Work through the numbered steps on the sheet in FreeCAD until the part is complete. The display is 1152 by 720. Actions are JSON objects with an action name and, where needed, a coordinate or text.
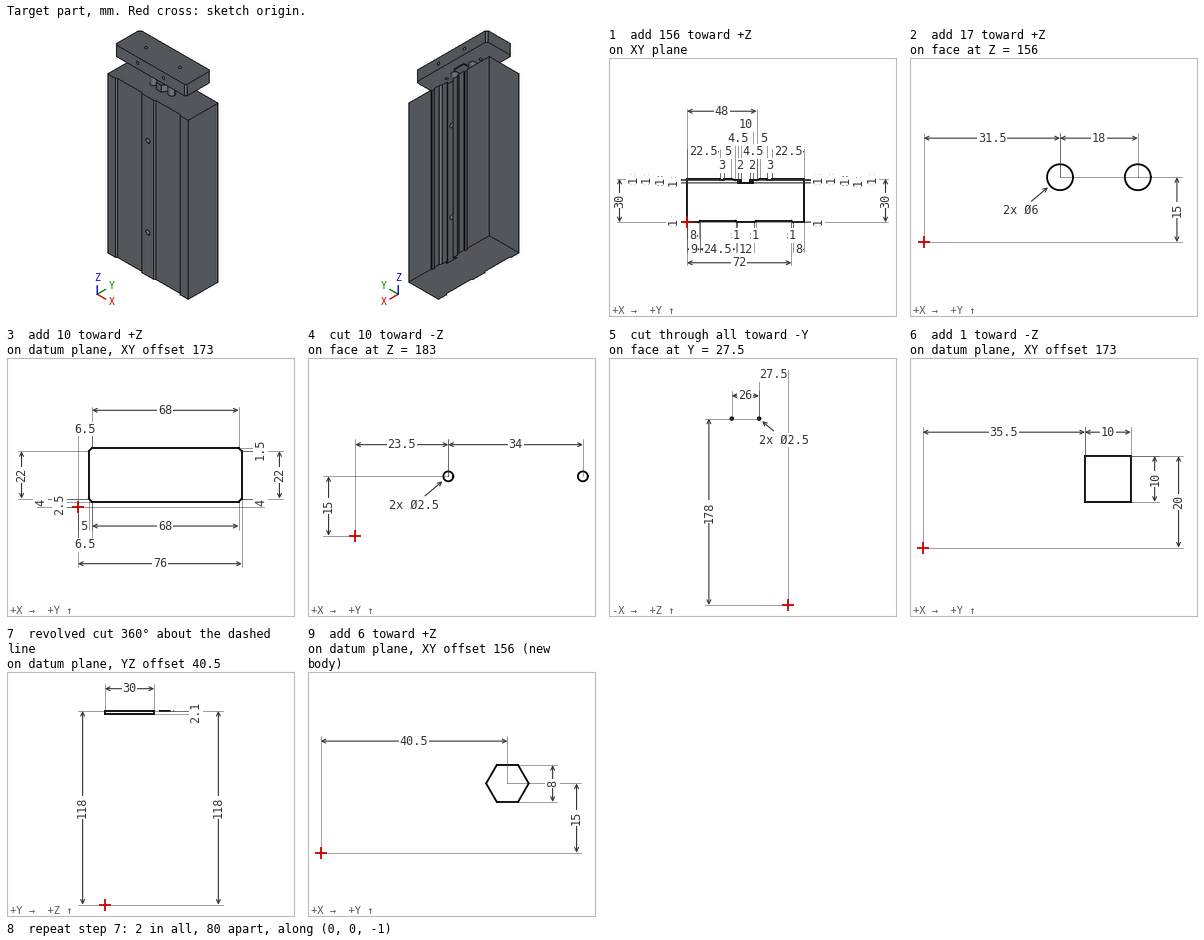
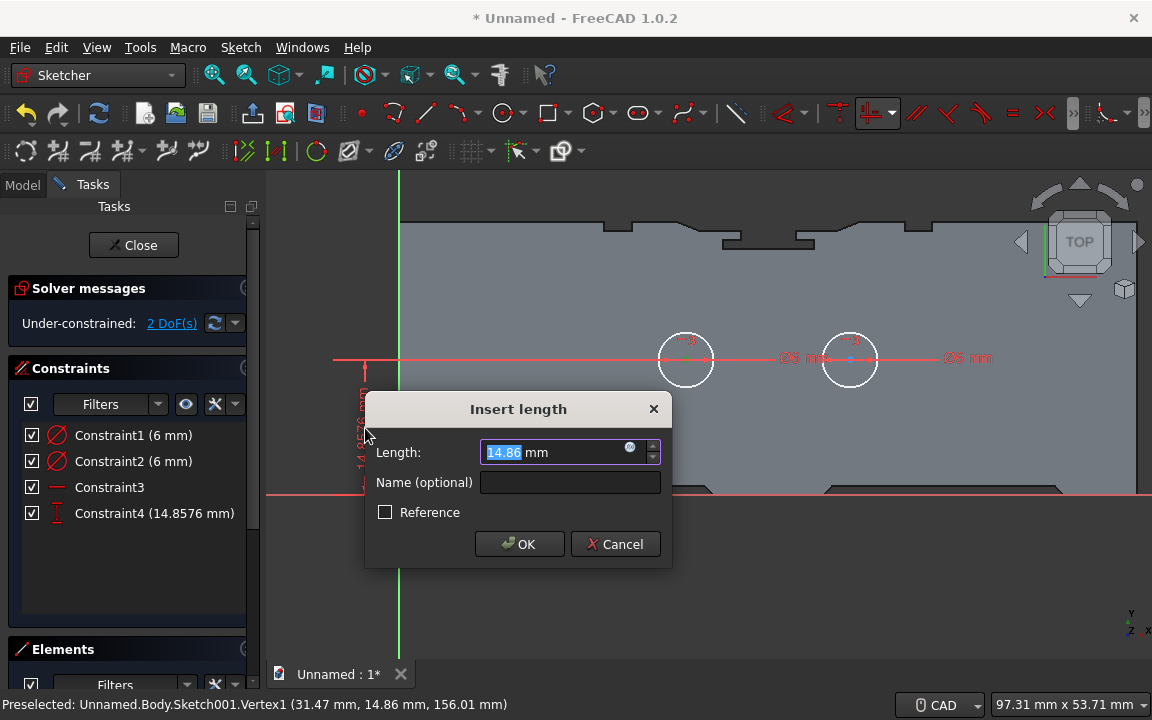
{"action": "type", "text": "15"}
{"action": "key", "text": "Return"}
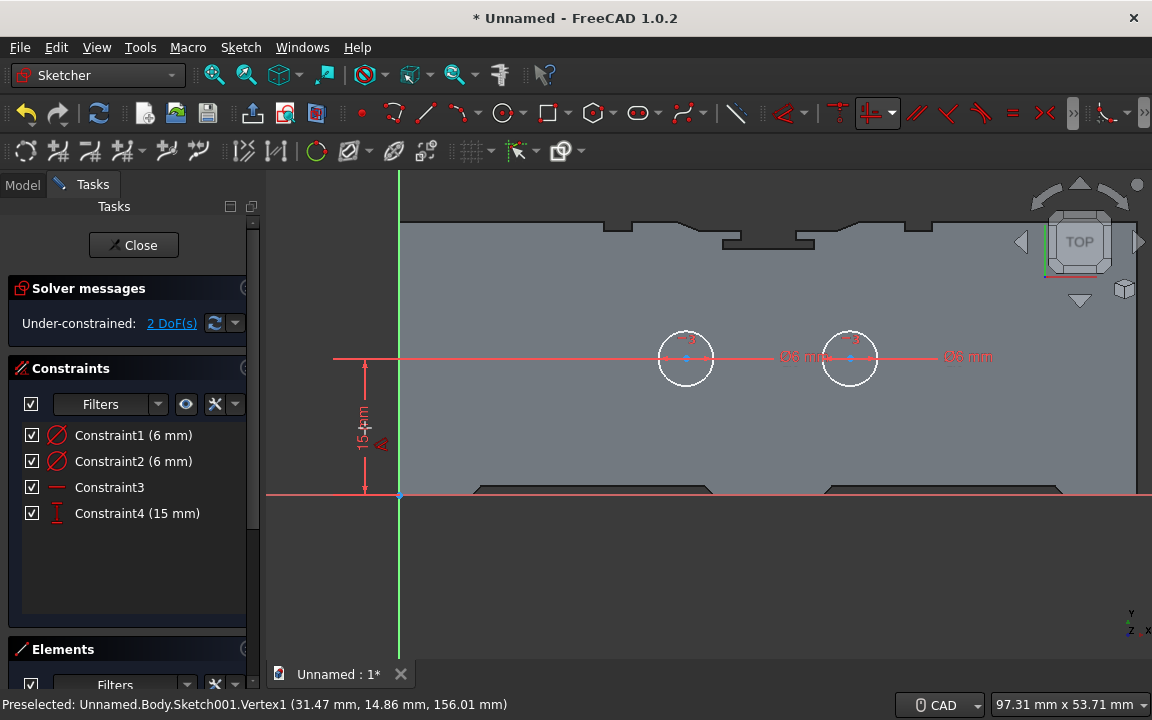
{"action": "left_click", "coordinate": [686, 359]}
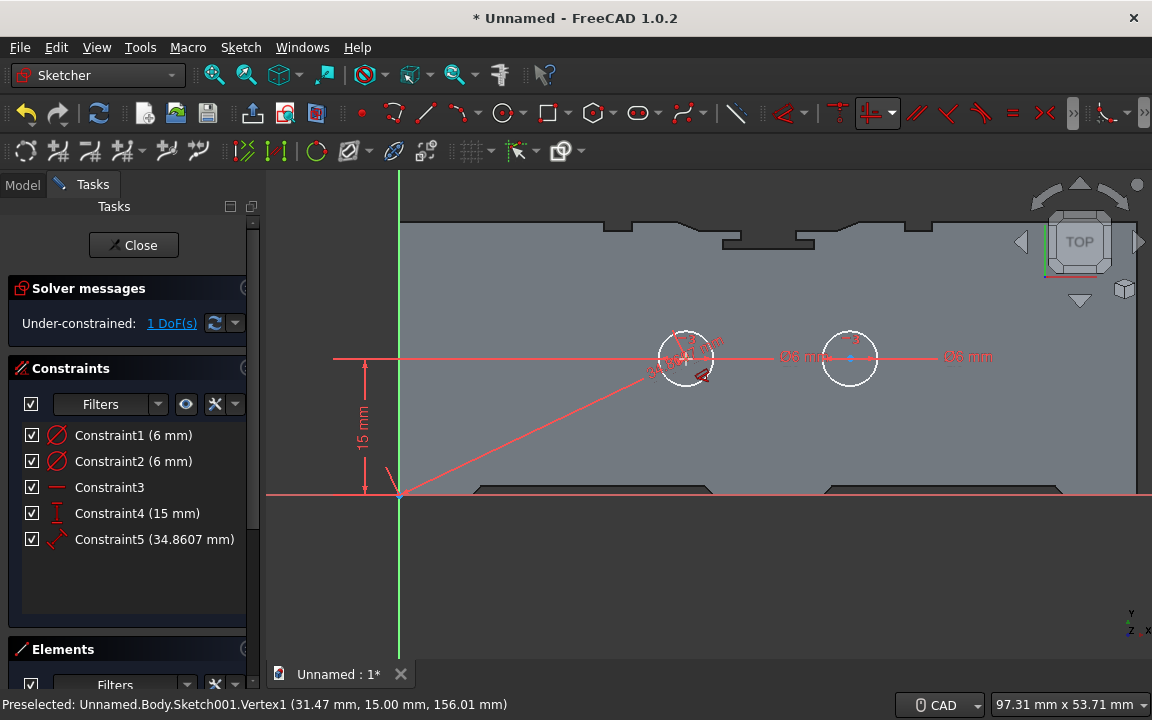
{"action": "left_click", "coordinate": [850, 359]}
{"action": "left_click", "coordinate": [768, 325]}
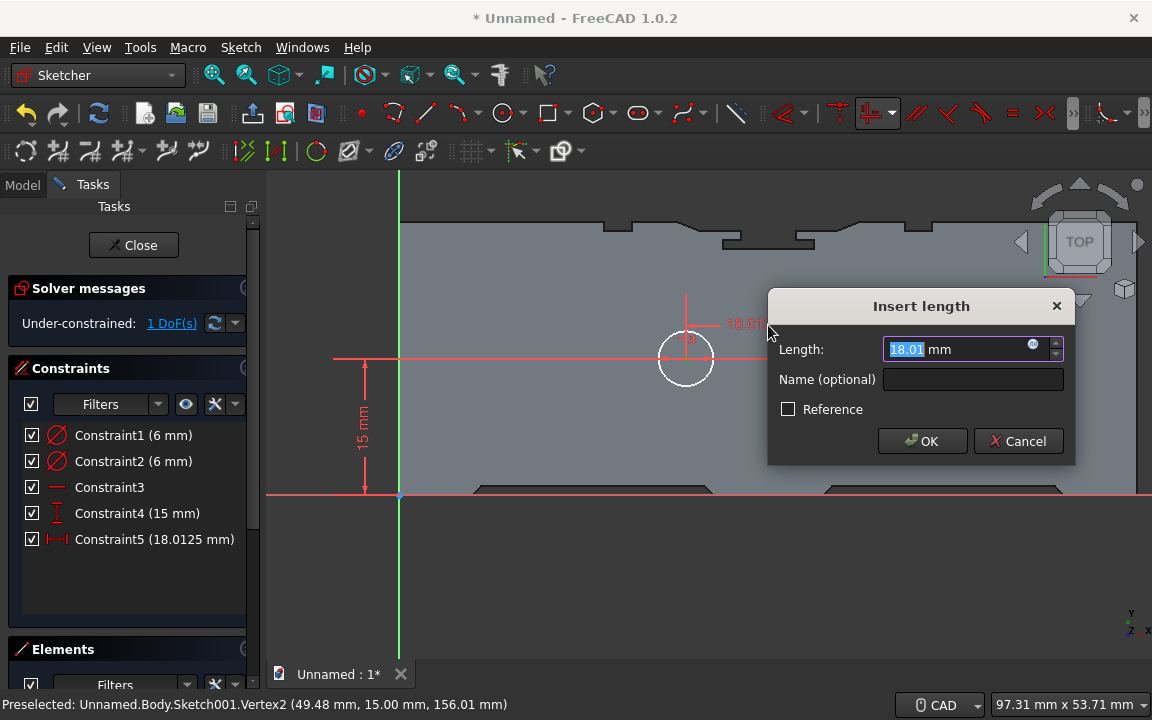
{"action": "type", "text": "18"}
{"action": "key", "text": "Return"}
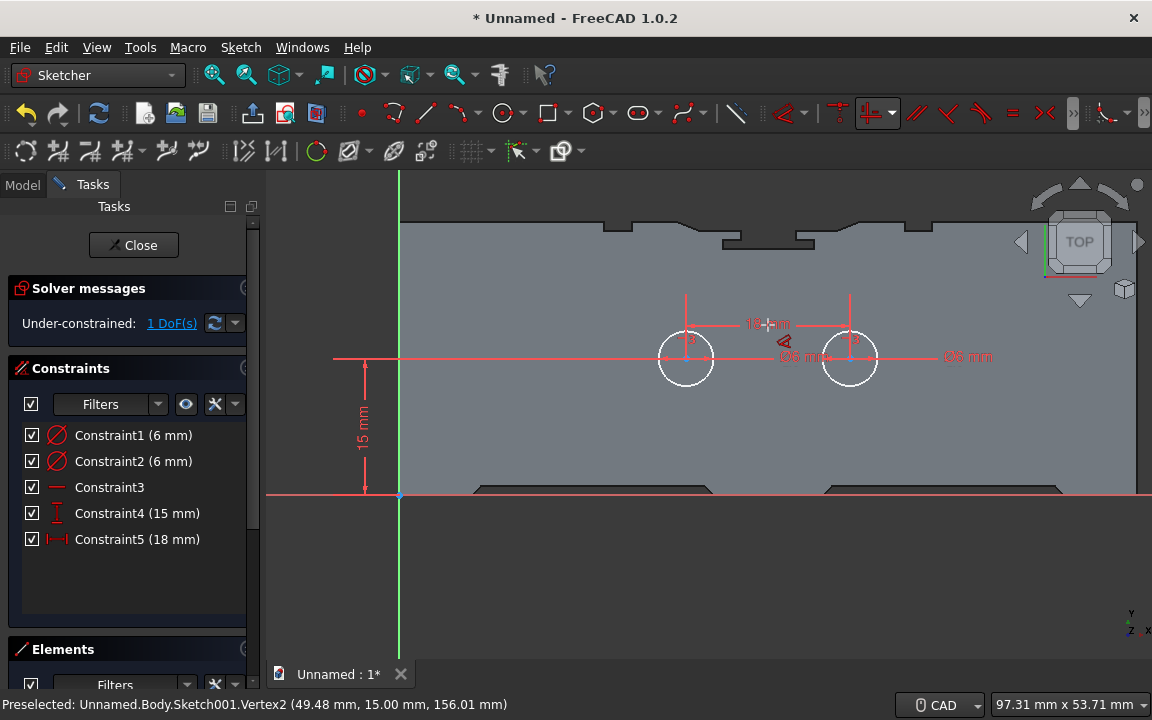
{"action": "left_click", "coordinate": [686, 359]}
{"action": "left_click", "coordinate": [543, 529]}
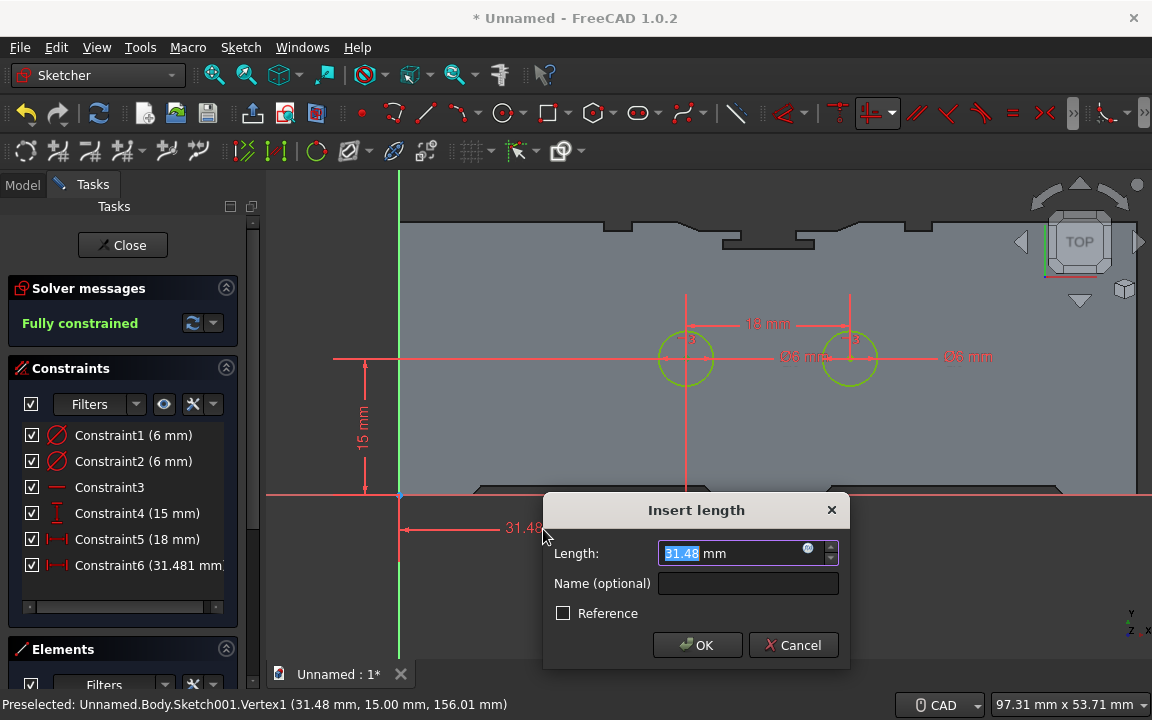
{"action": "type", "text": "31.5"}
{"action": "key", "text": "Return"}
{"action": "key", "text": "Escape"}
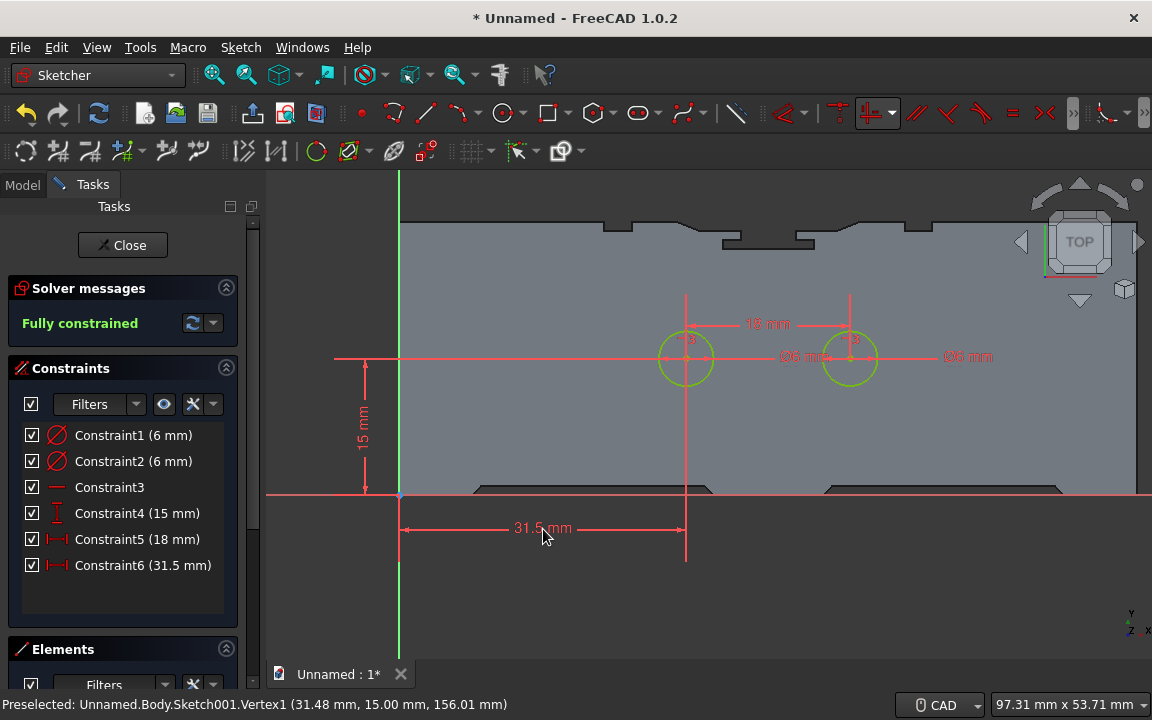
{"action": "left_click", "coordinate": [123, 245]}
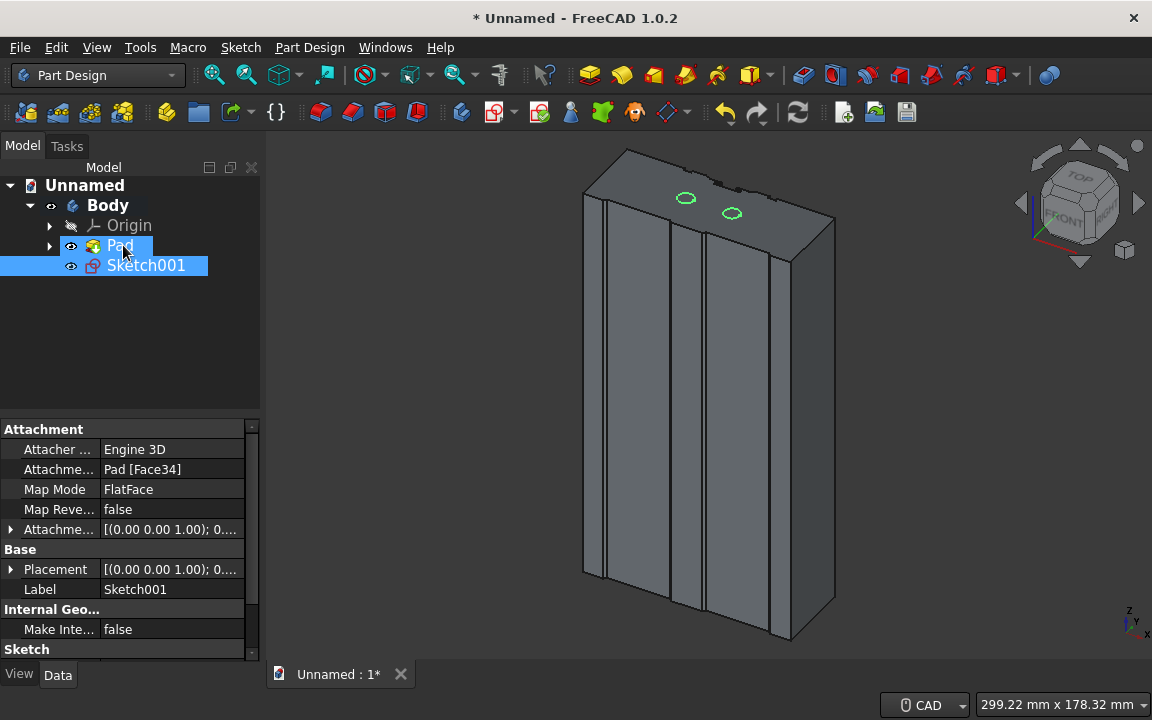
{"action": "left_click", "coordinate": [590, 76]}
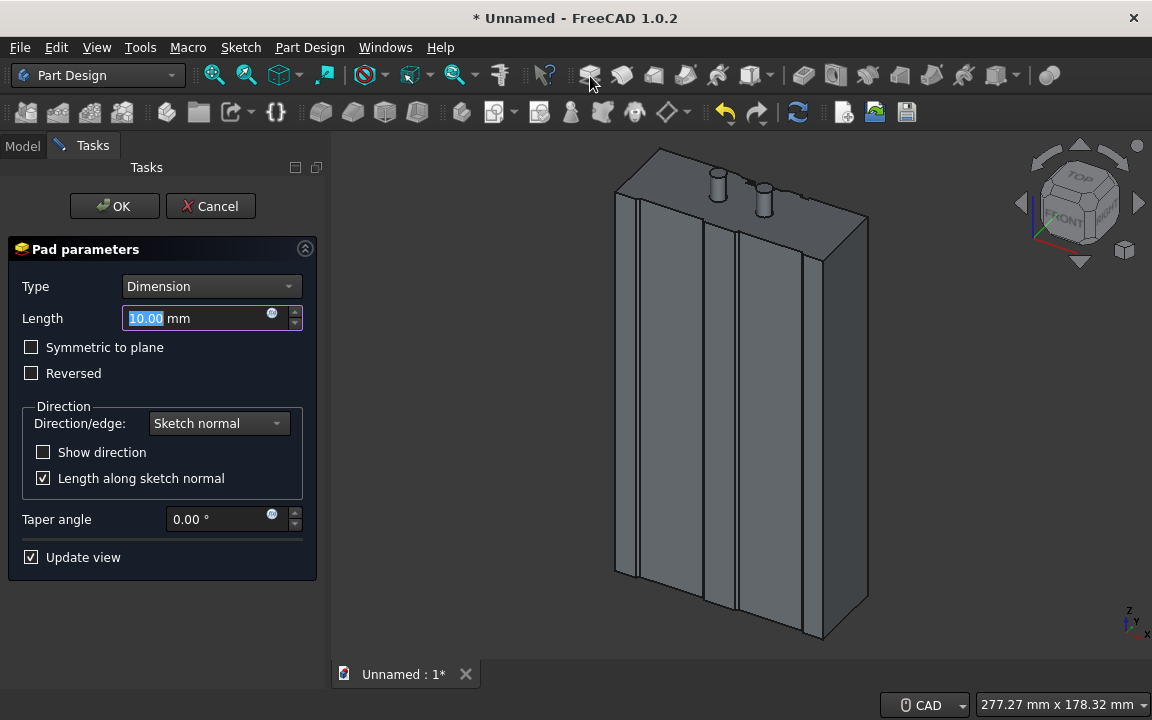
{"action": "type", "text": "17"}
{"action": "key", "text": "Tab"}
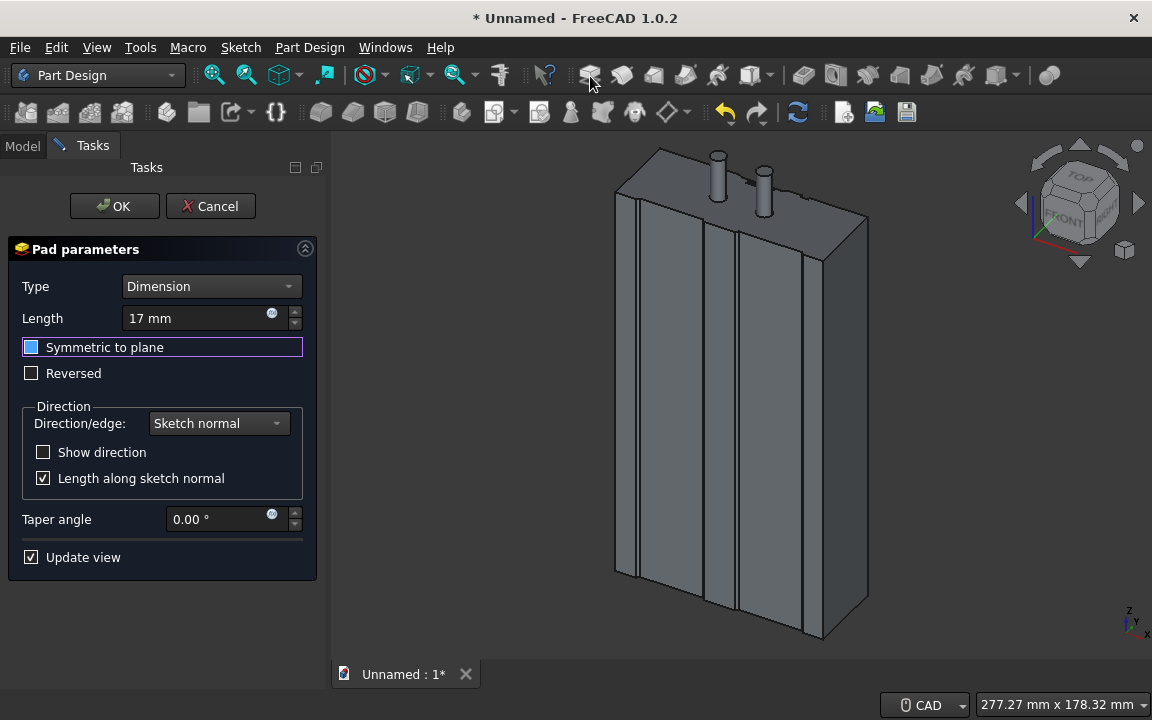
{"action": "left_click", "coordinate": [115, 206]}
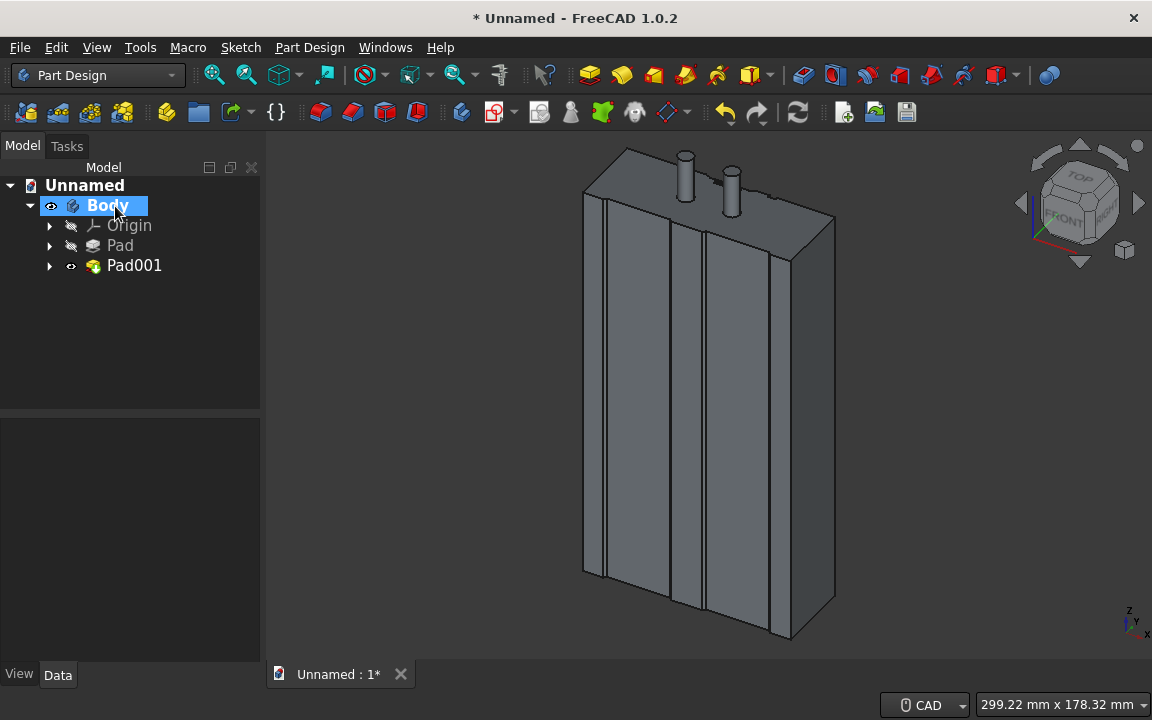
{"action": "key", "text": "v f"}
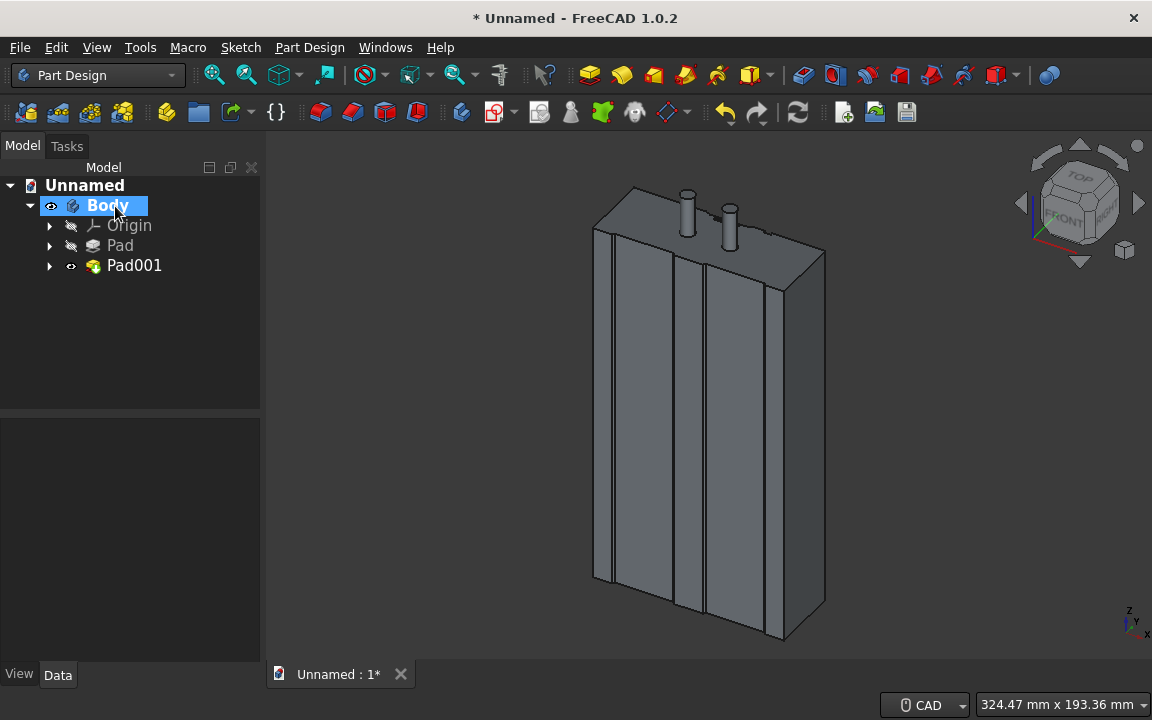
{"action": "key", "text": "0"}